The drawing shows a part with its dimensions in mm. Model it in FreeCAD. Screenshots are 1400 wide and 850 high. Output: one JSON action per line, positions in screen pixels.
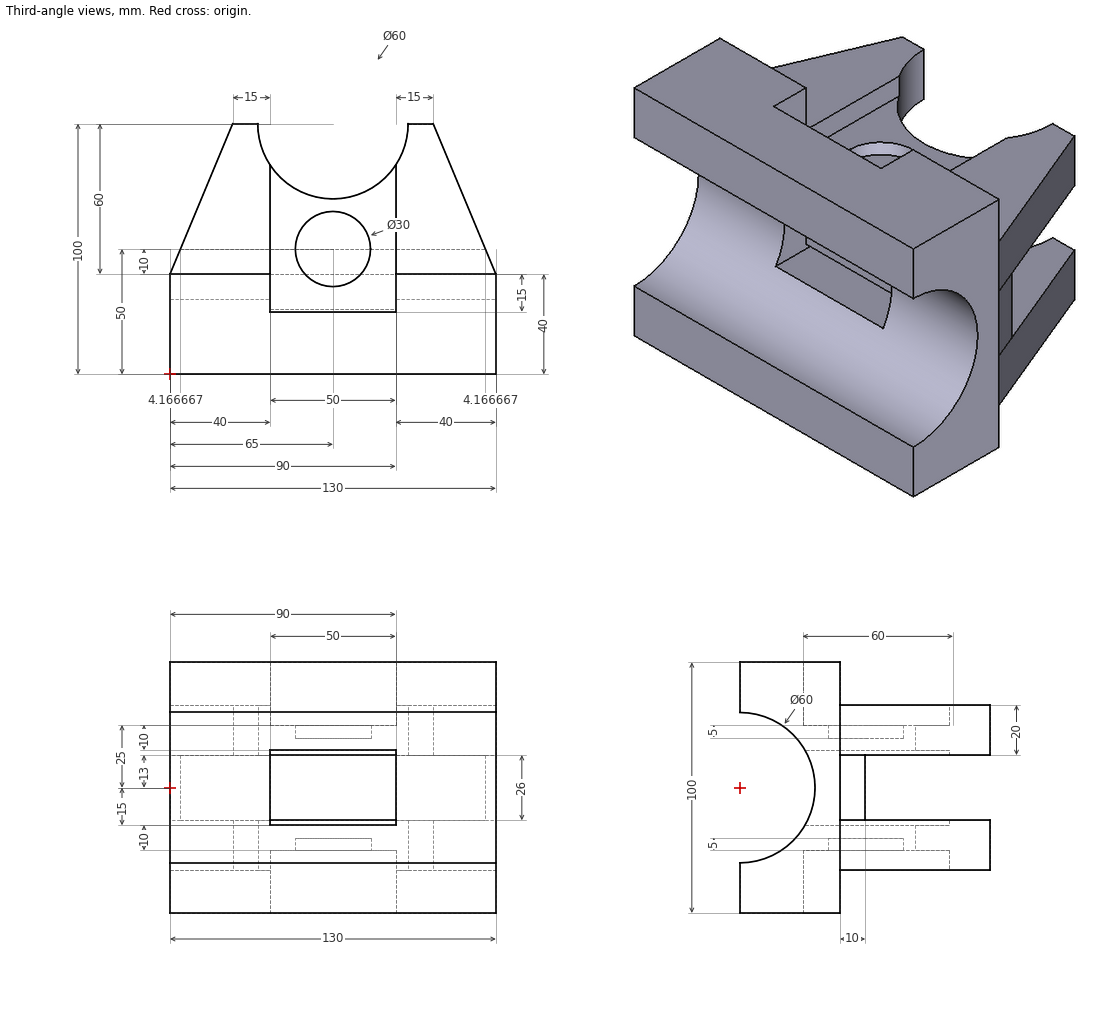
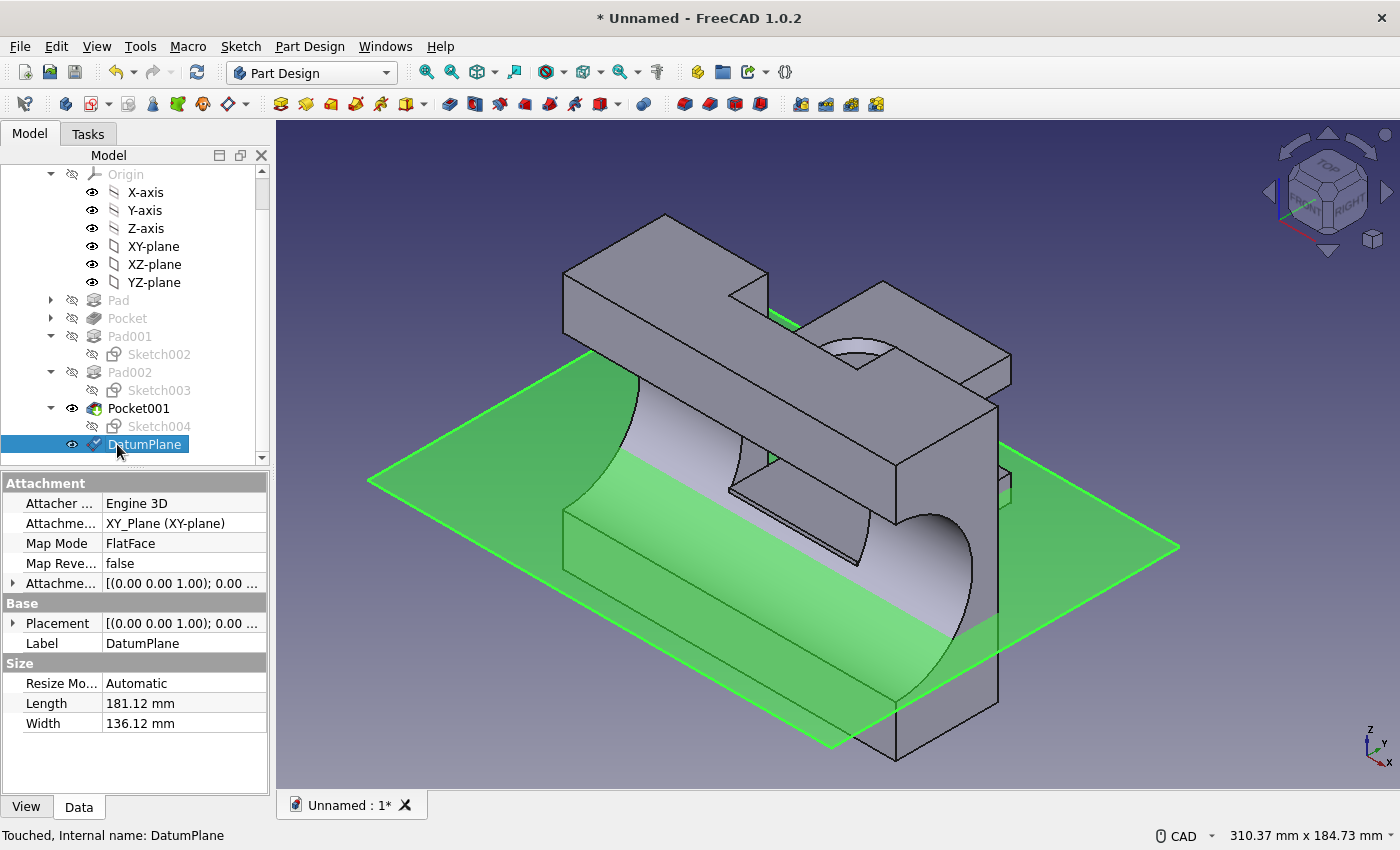
{"action": "left_click", "coordinate": [90, 104]}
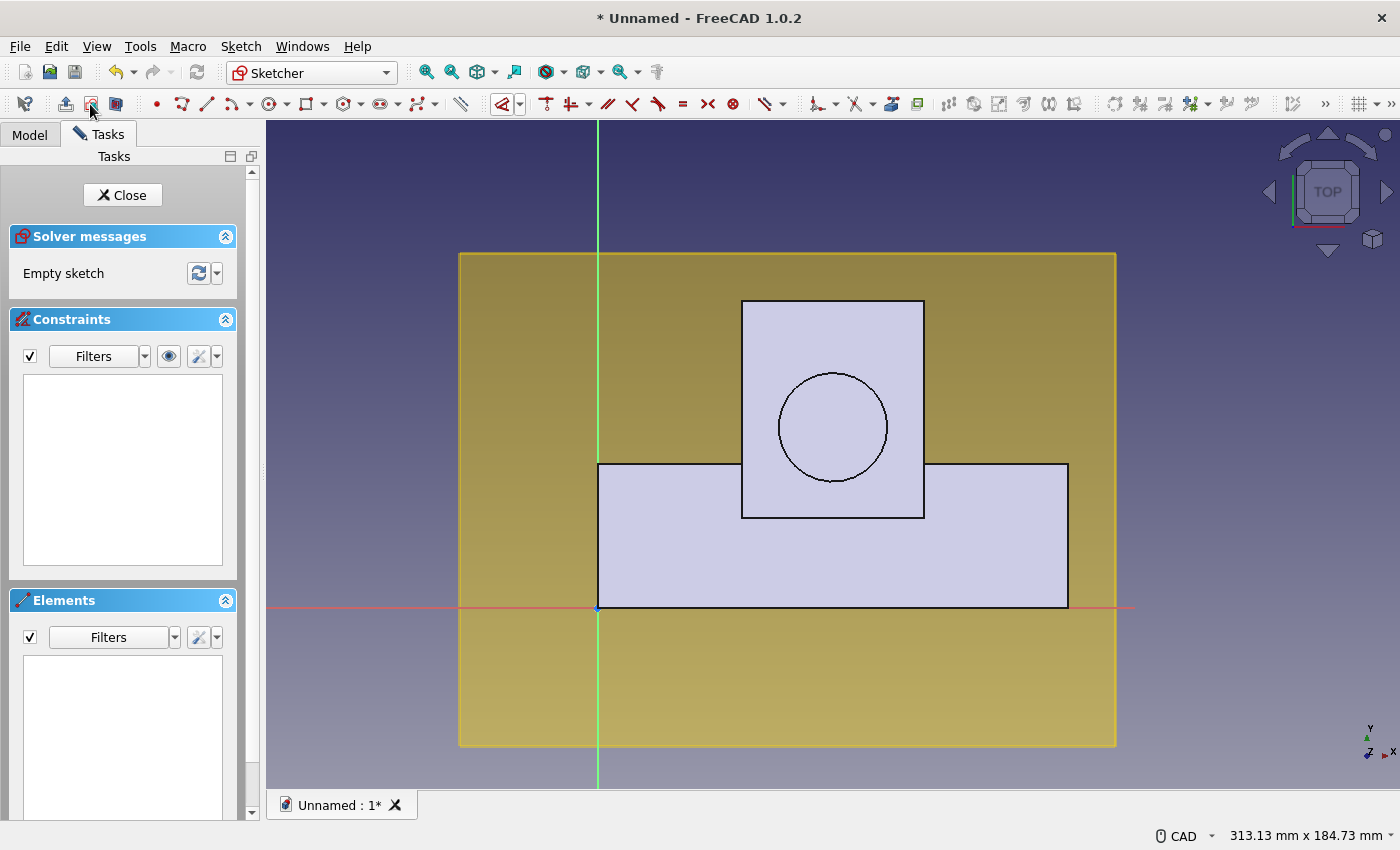
{"action": "left_click", "coordinate": [116, 104]}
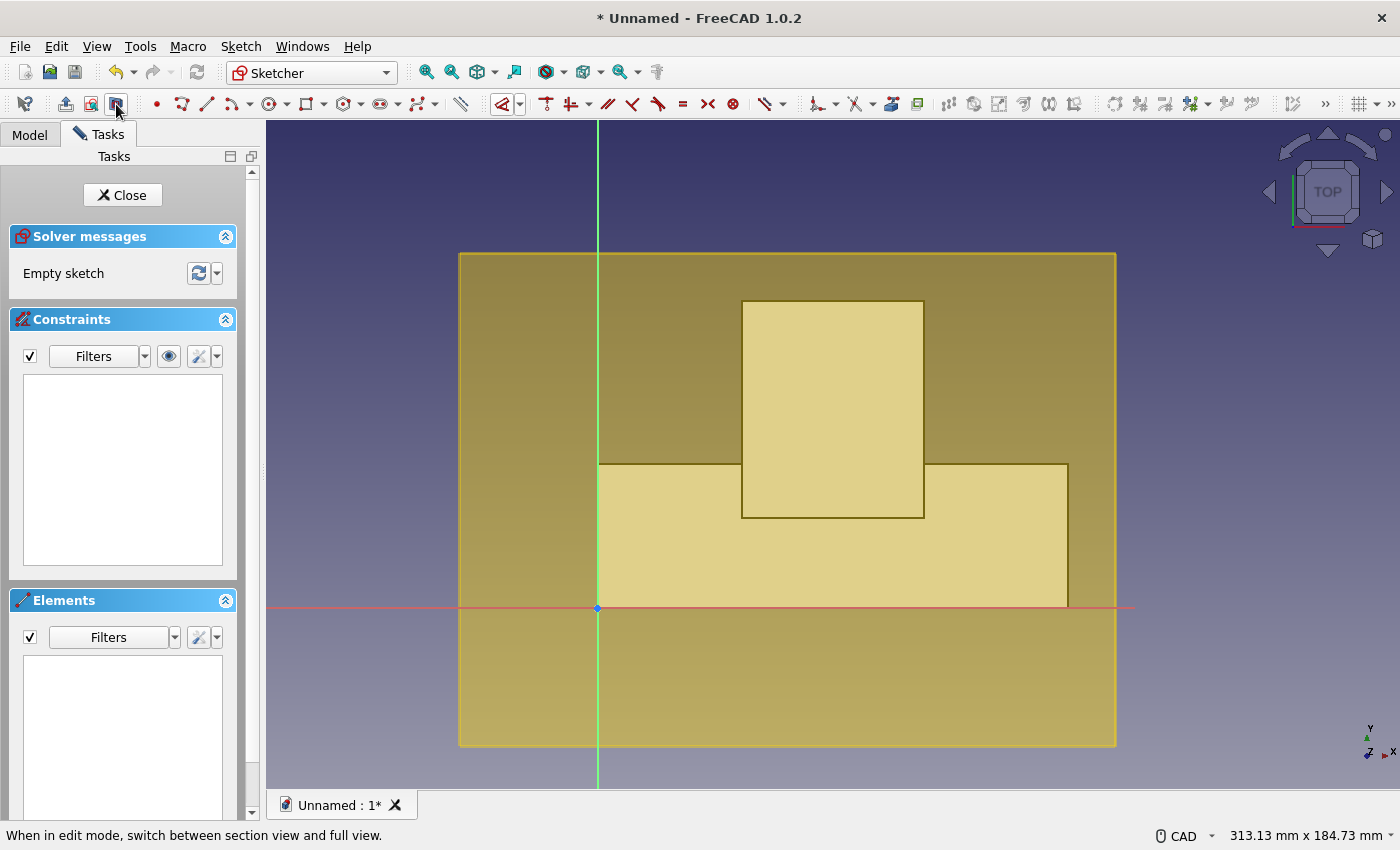
{"action": "scroll", "coordinate": [855, 418], "scroll_direction": "up", "scroll_amount": 7}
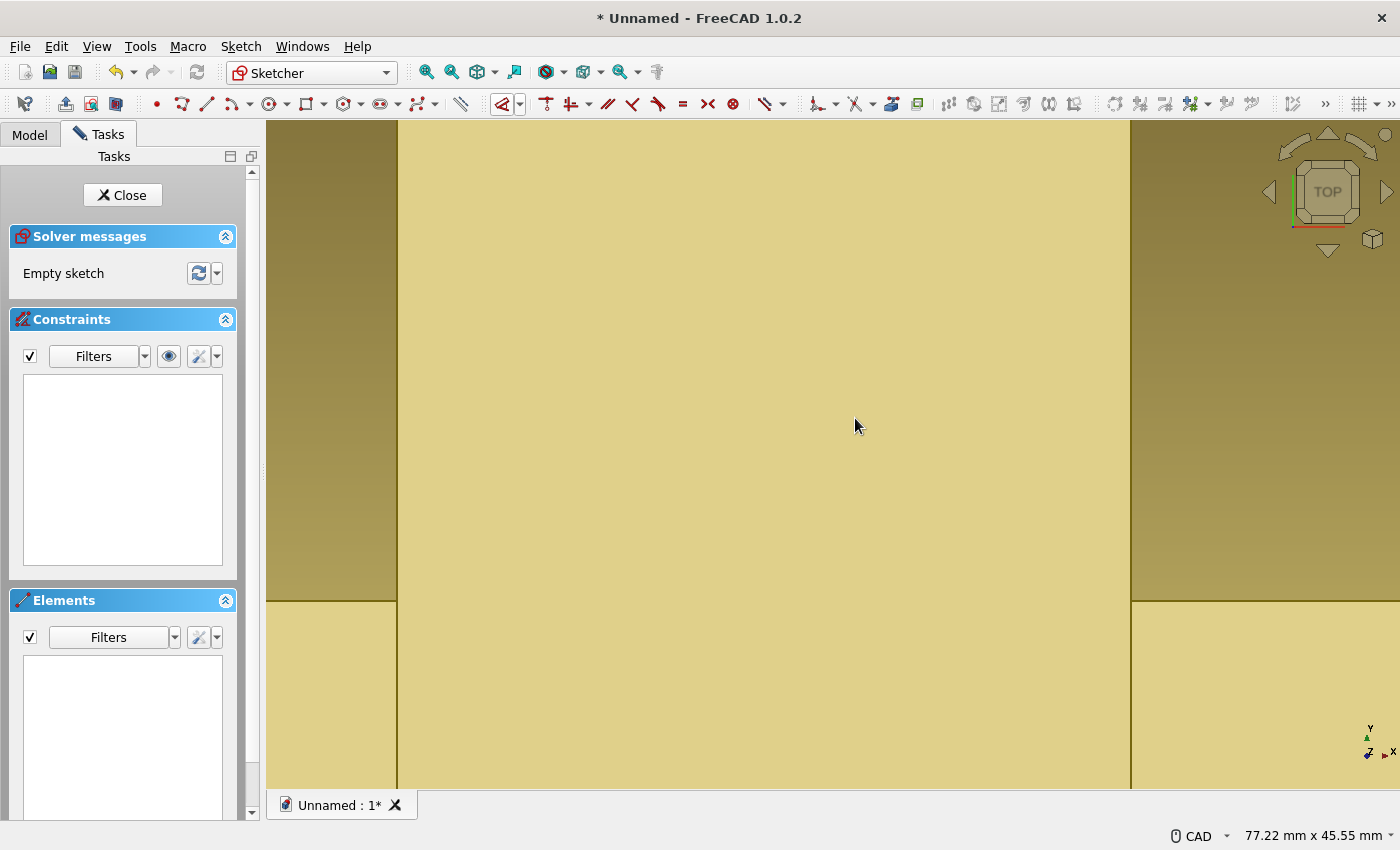
{"action": "left_click", "coordinate": [268, 104]}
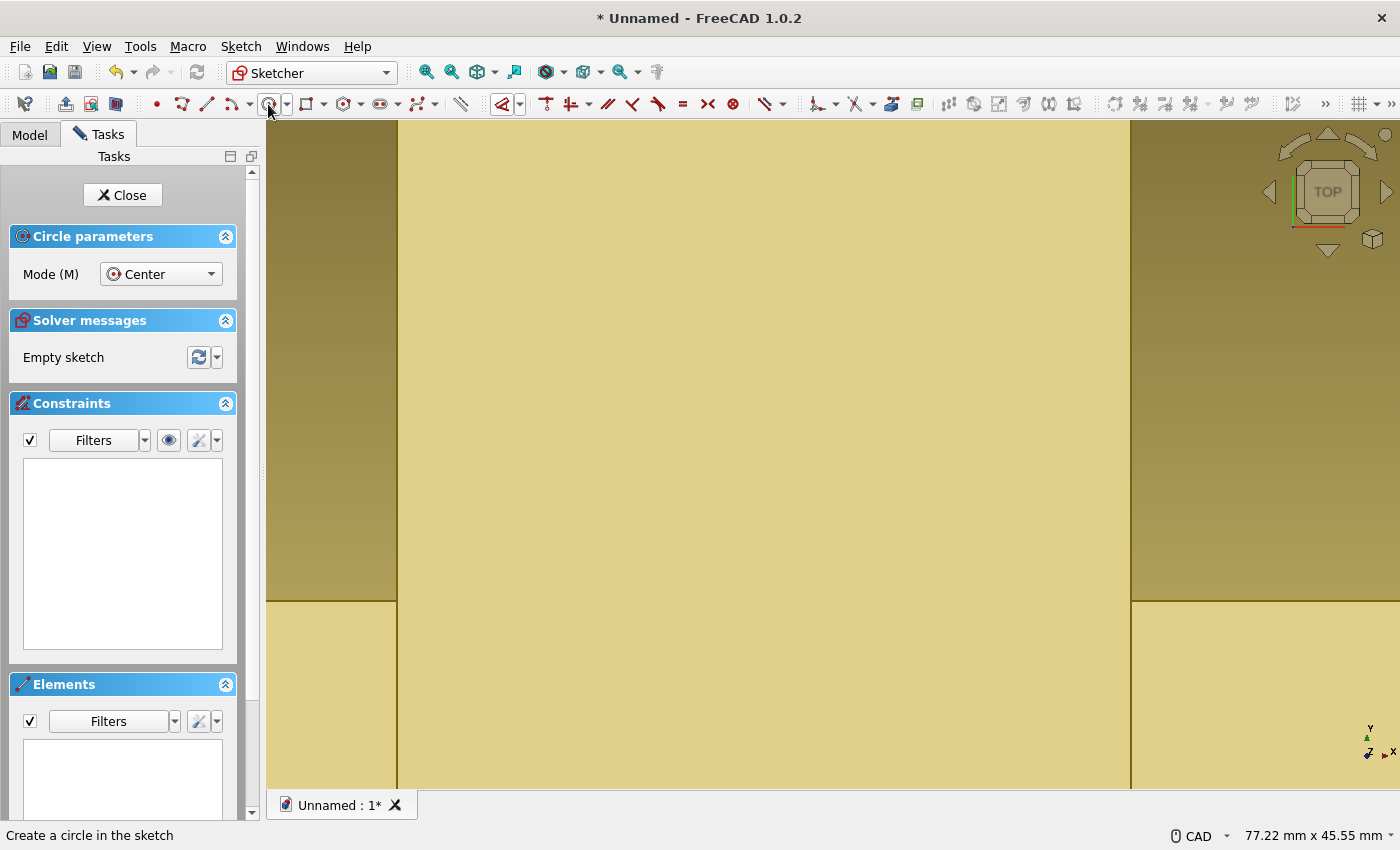
{"action": "left_click", "coordinate": [764, 455]}
{"action": "mouse_move", "coordinate": [920, 299]}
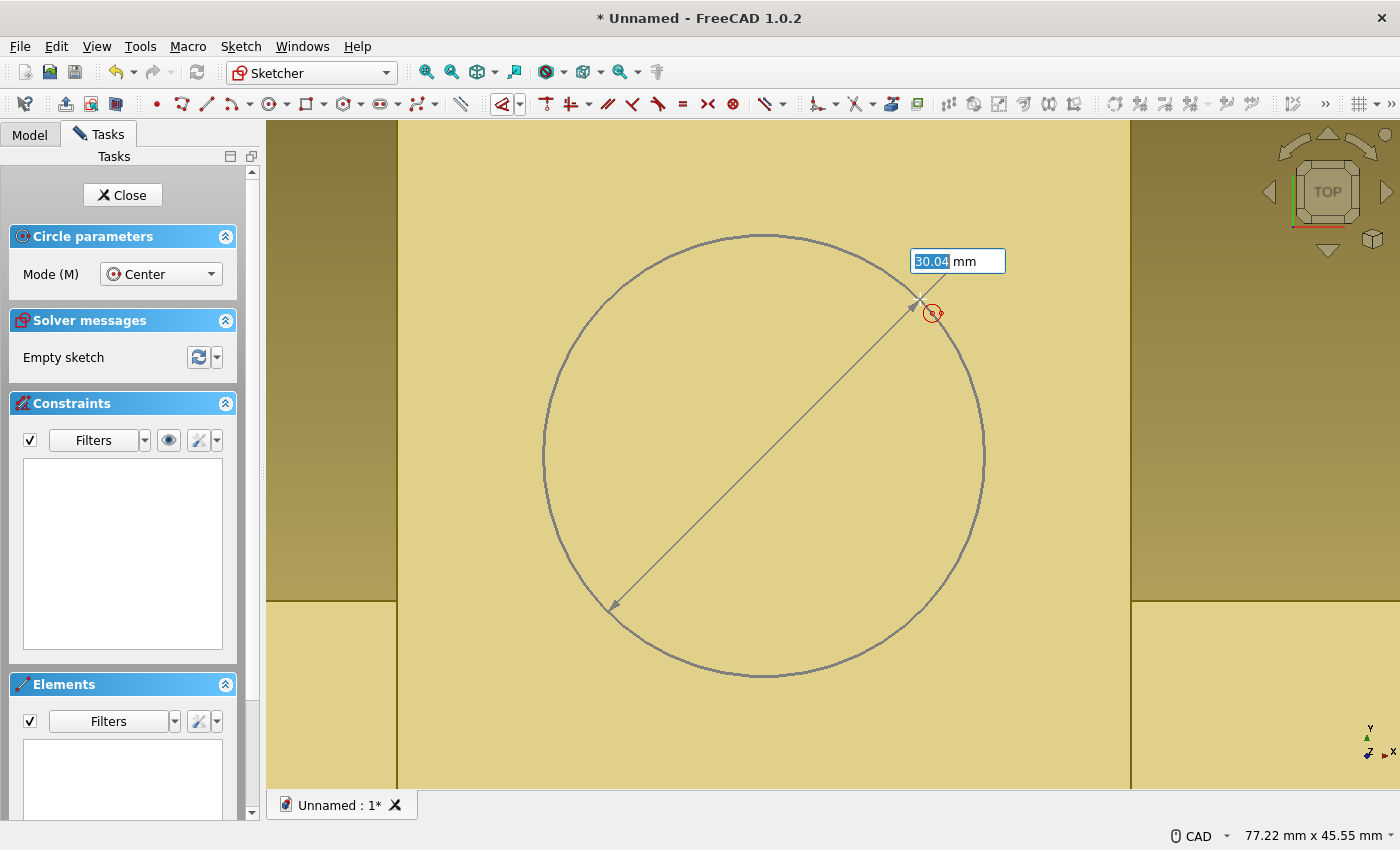
{"action": "type", "text": "30"}
{"action": "key", "text": "Return"}
{"action": "key", "text": "Escape"}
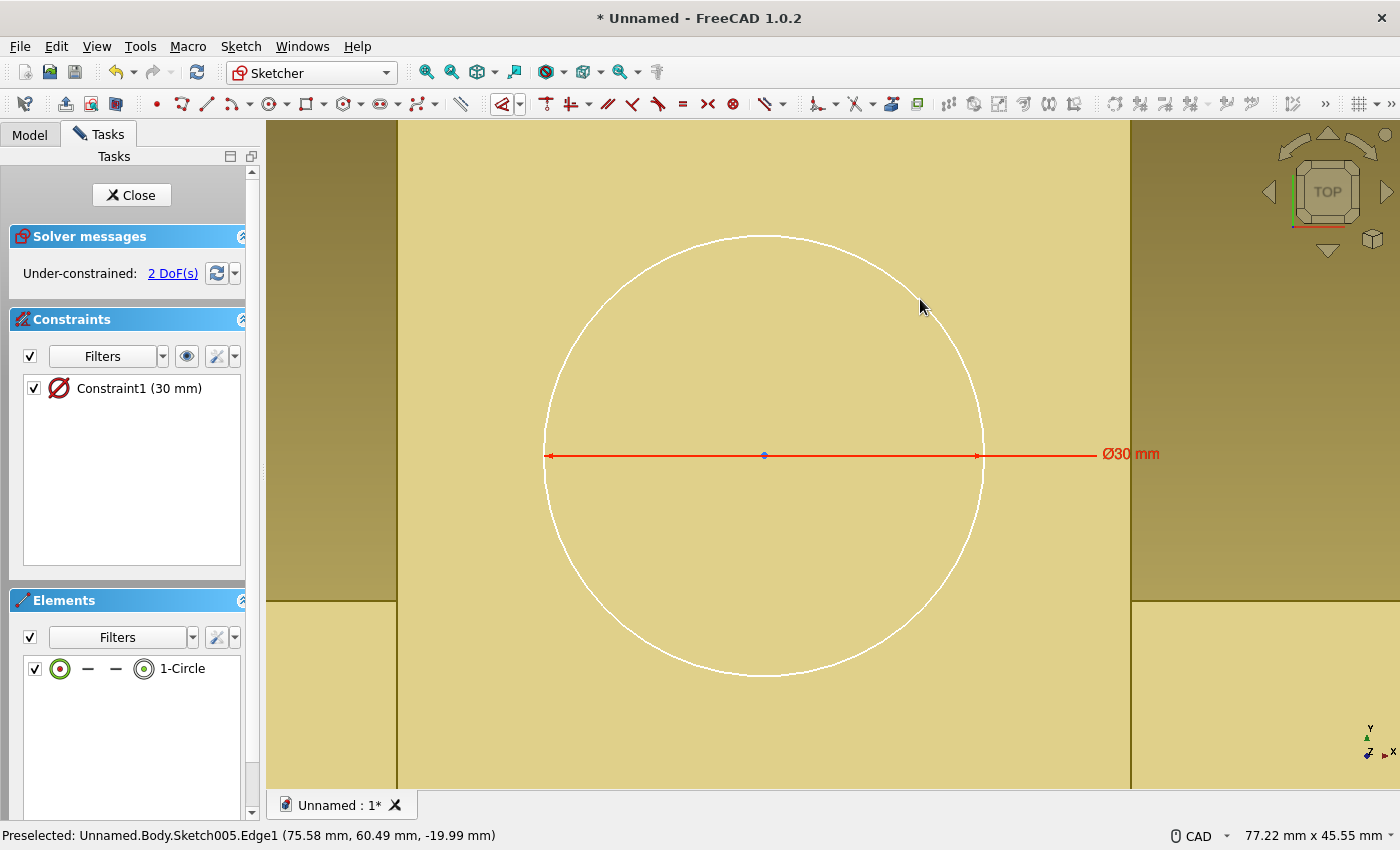
{"action": "left_click", "coordinate": [764, 456]}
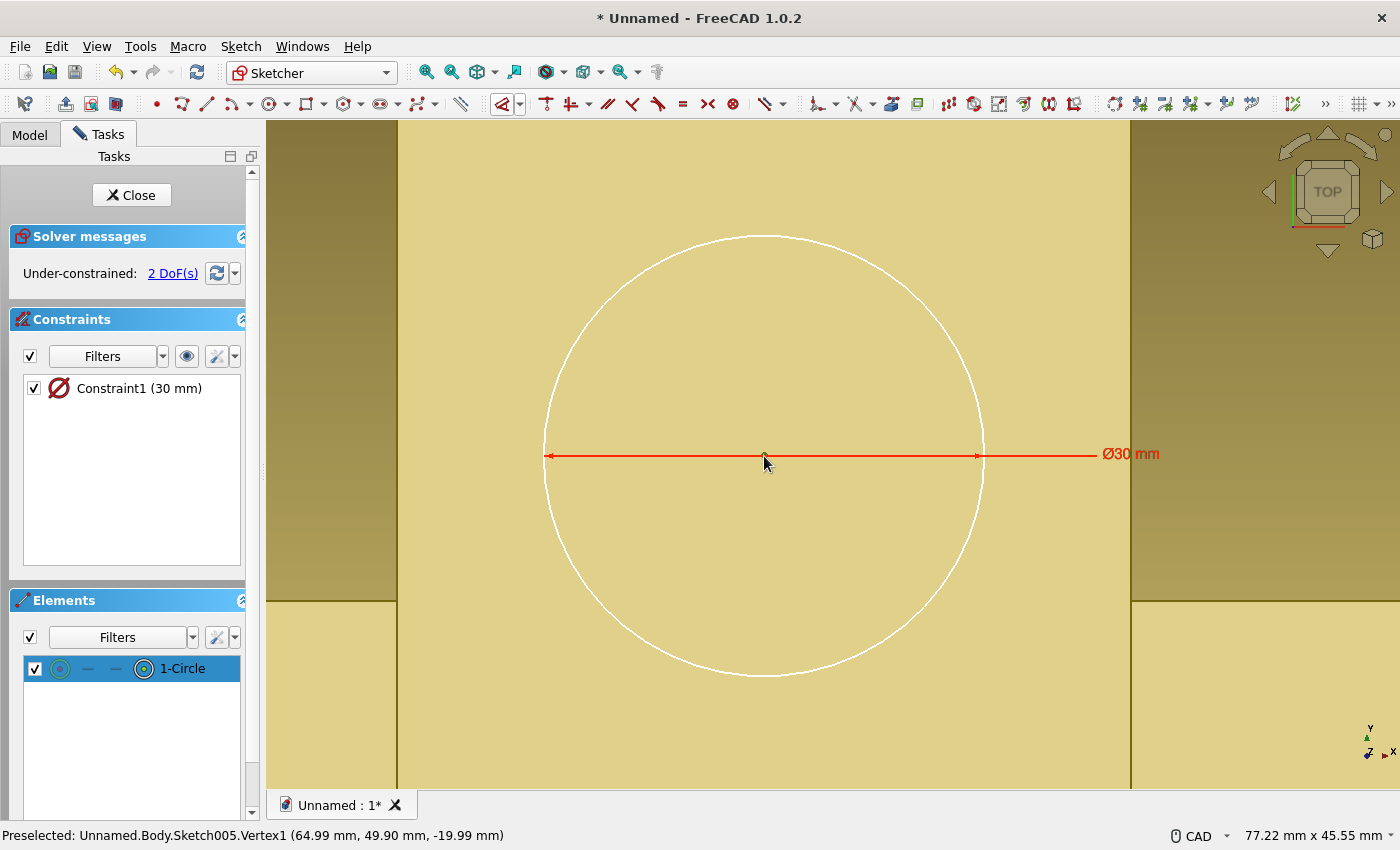
{"action": "key", "text": "l"}